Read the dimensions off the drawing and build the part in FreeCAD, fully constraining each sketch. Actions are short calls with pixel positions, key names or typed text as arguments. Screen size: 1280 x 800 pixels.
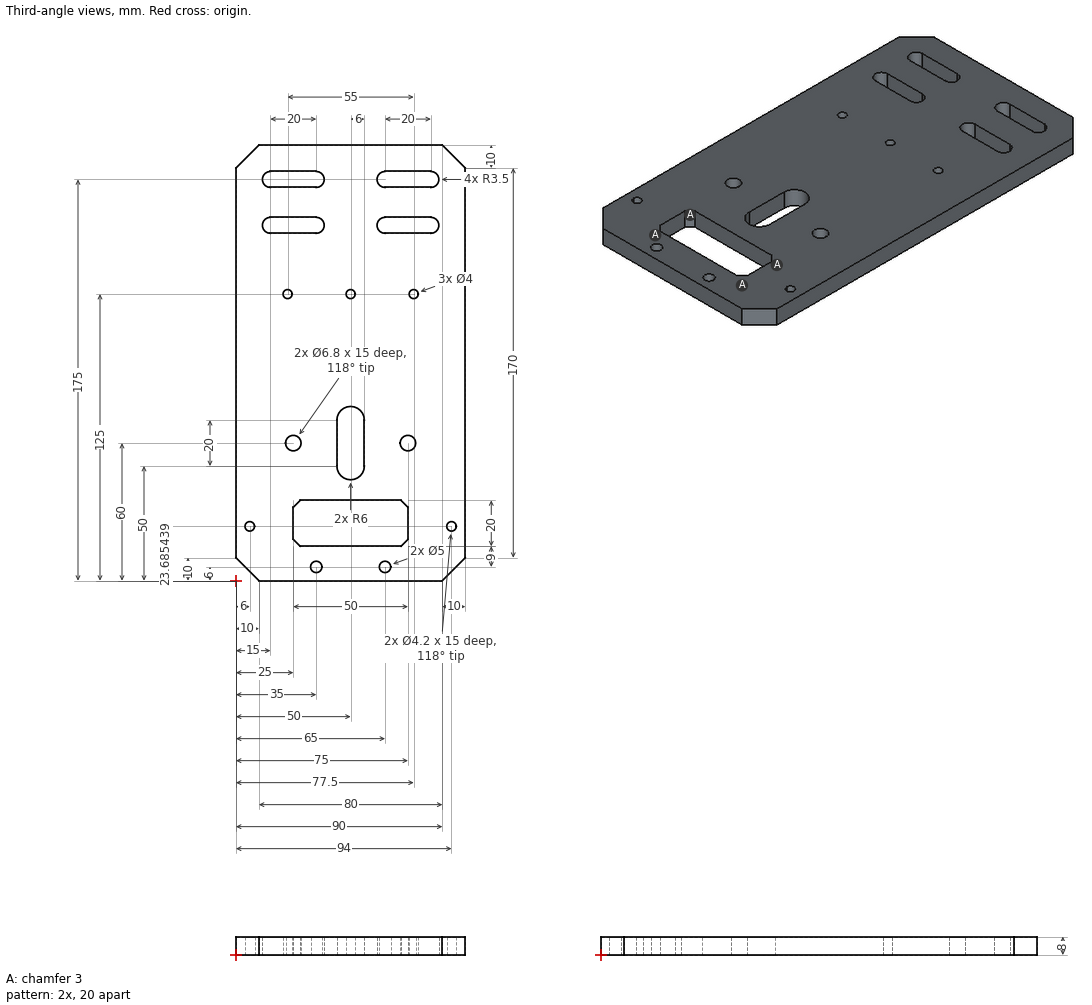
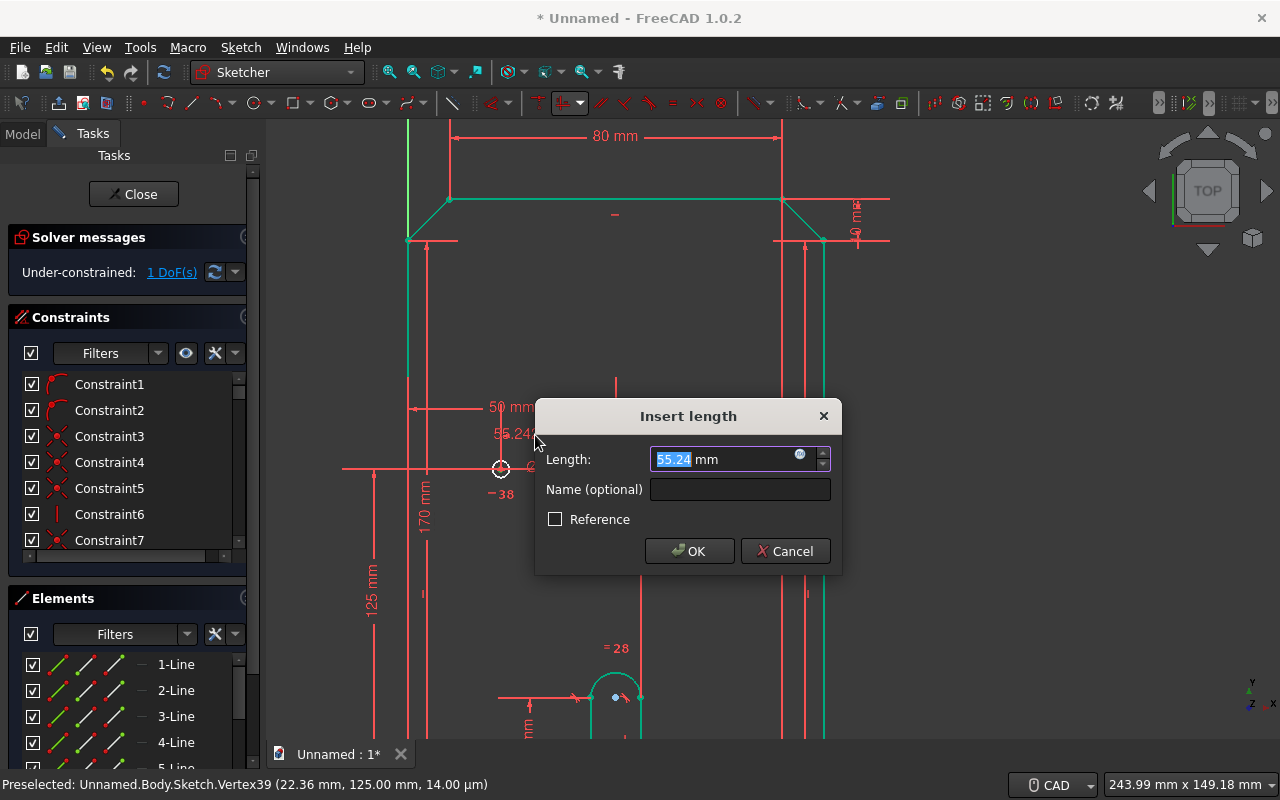
text(55)
key(Return)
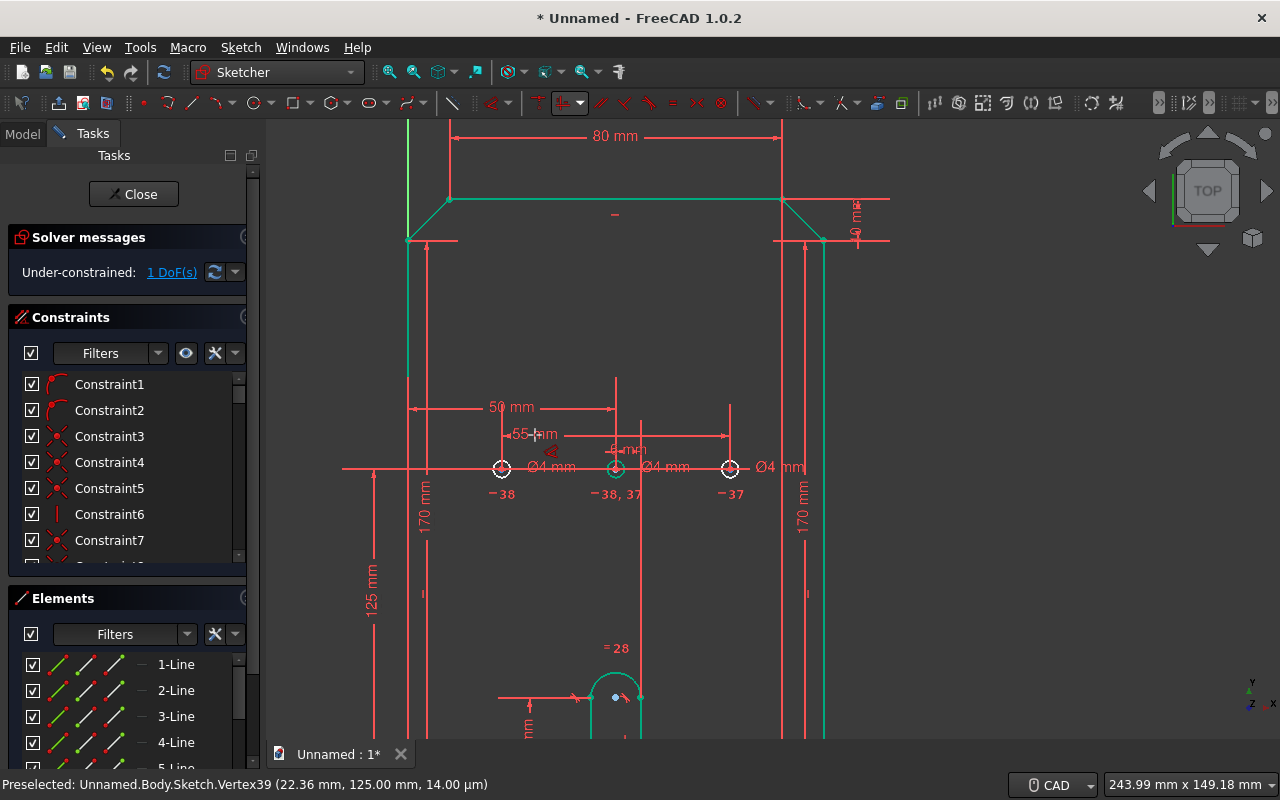
click(730, 469)
click(456, 435)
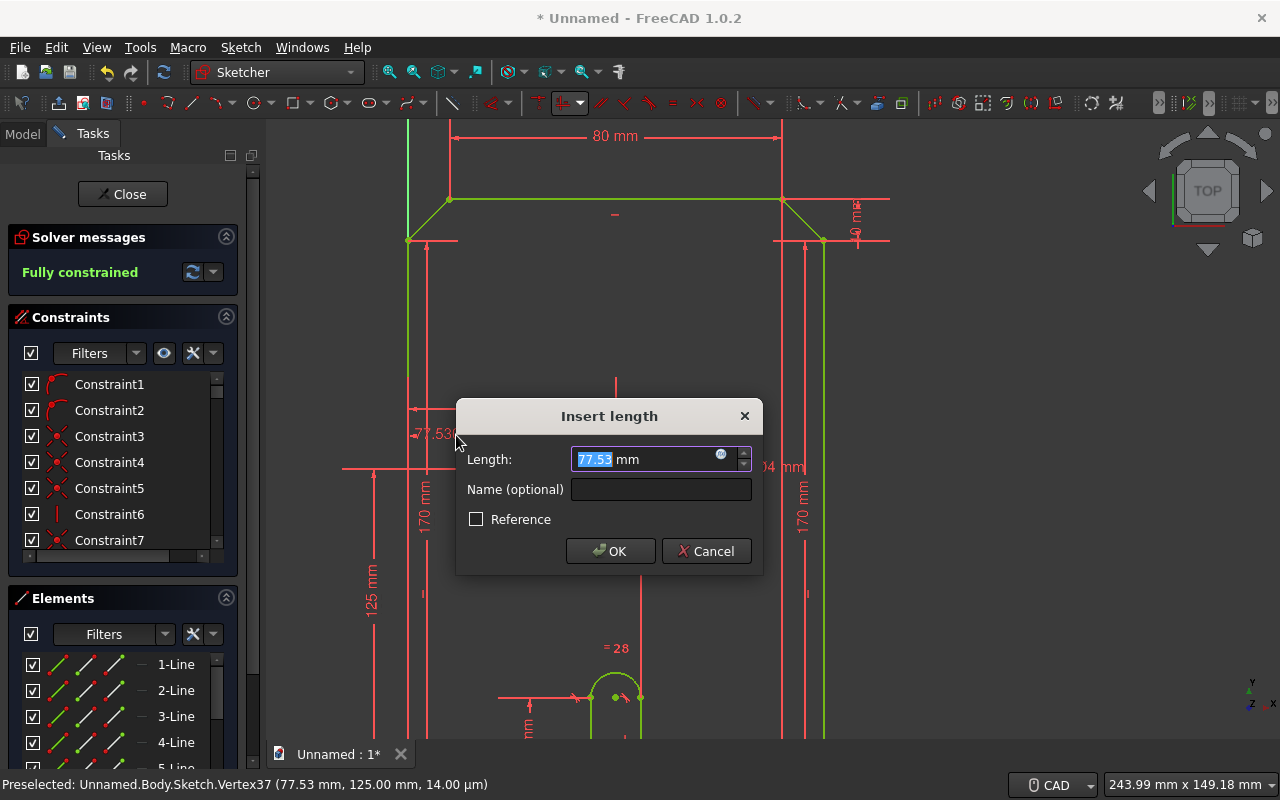
text(77.5)
key(Return)
key(Escape)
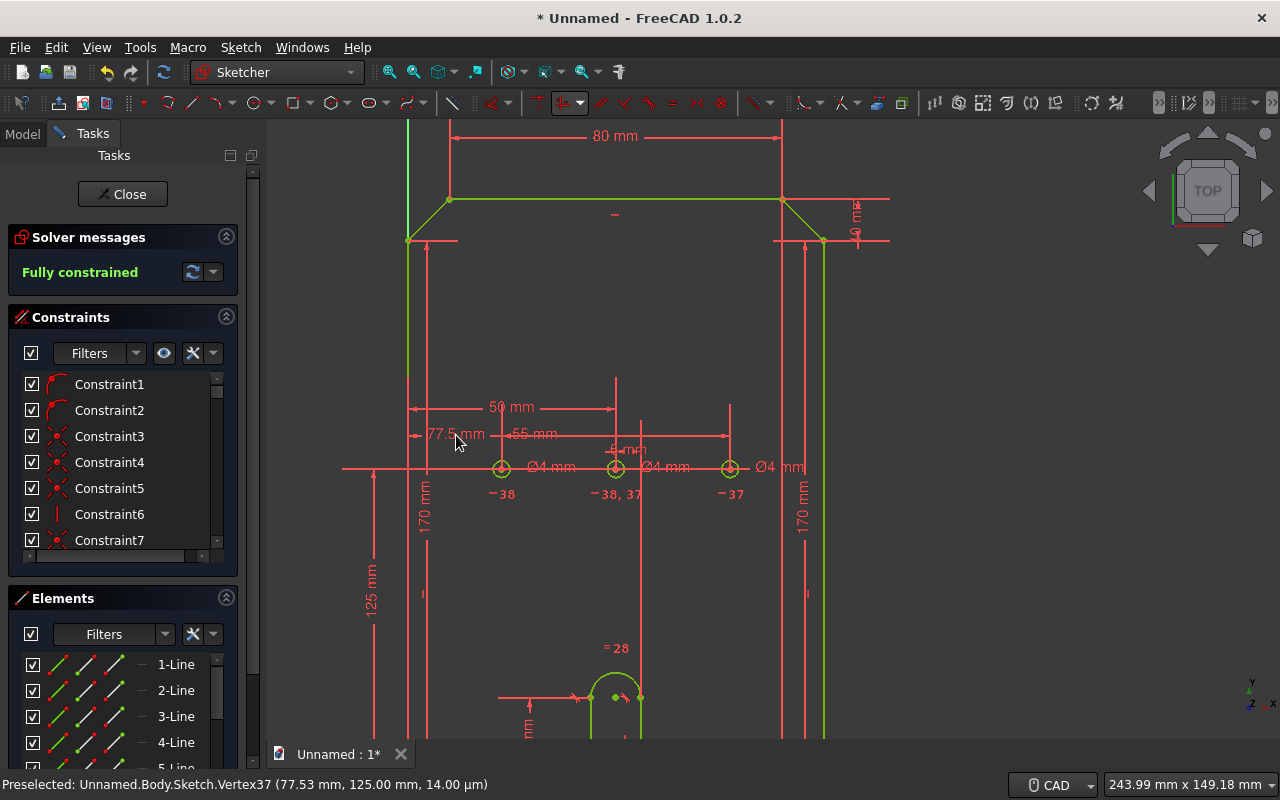
click(123, 194)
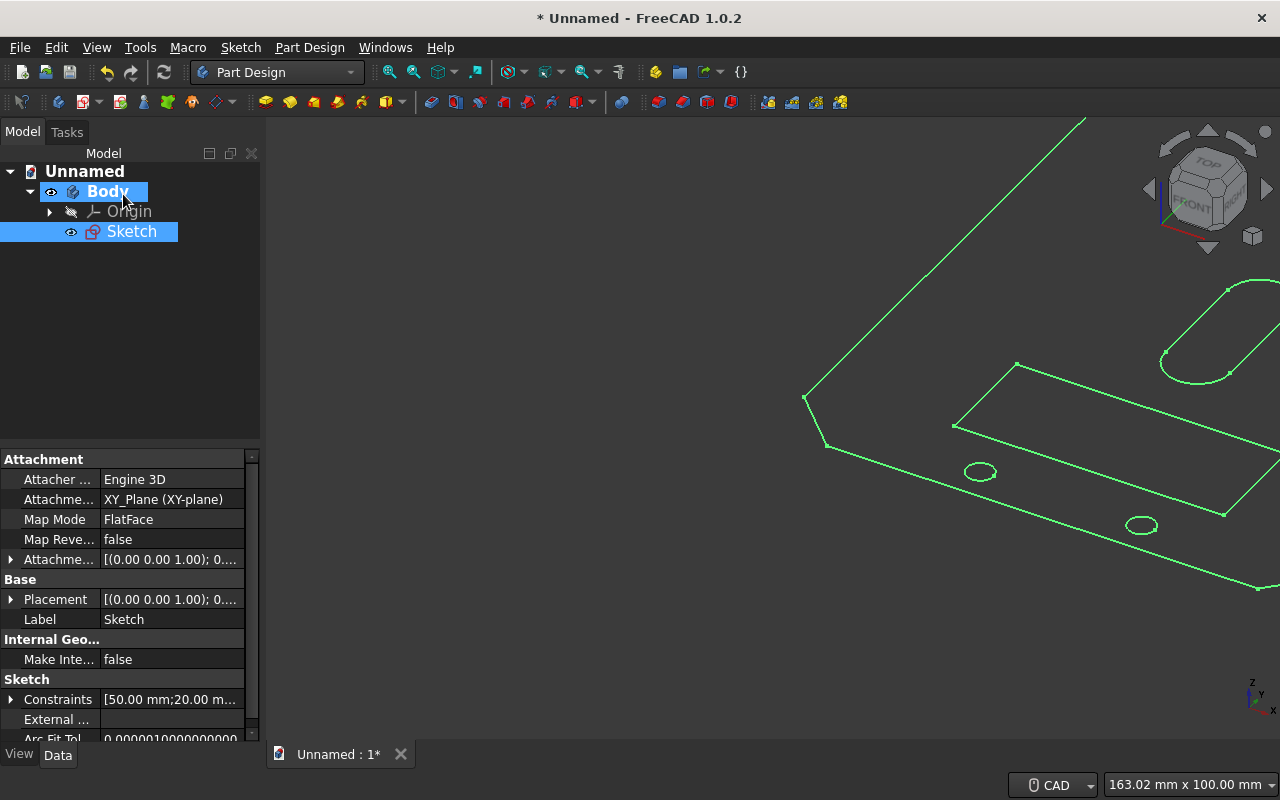
click(266, 102)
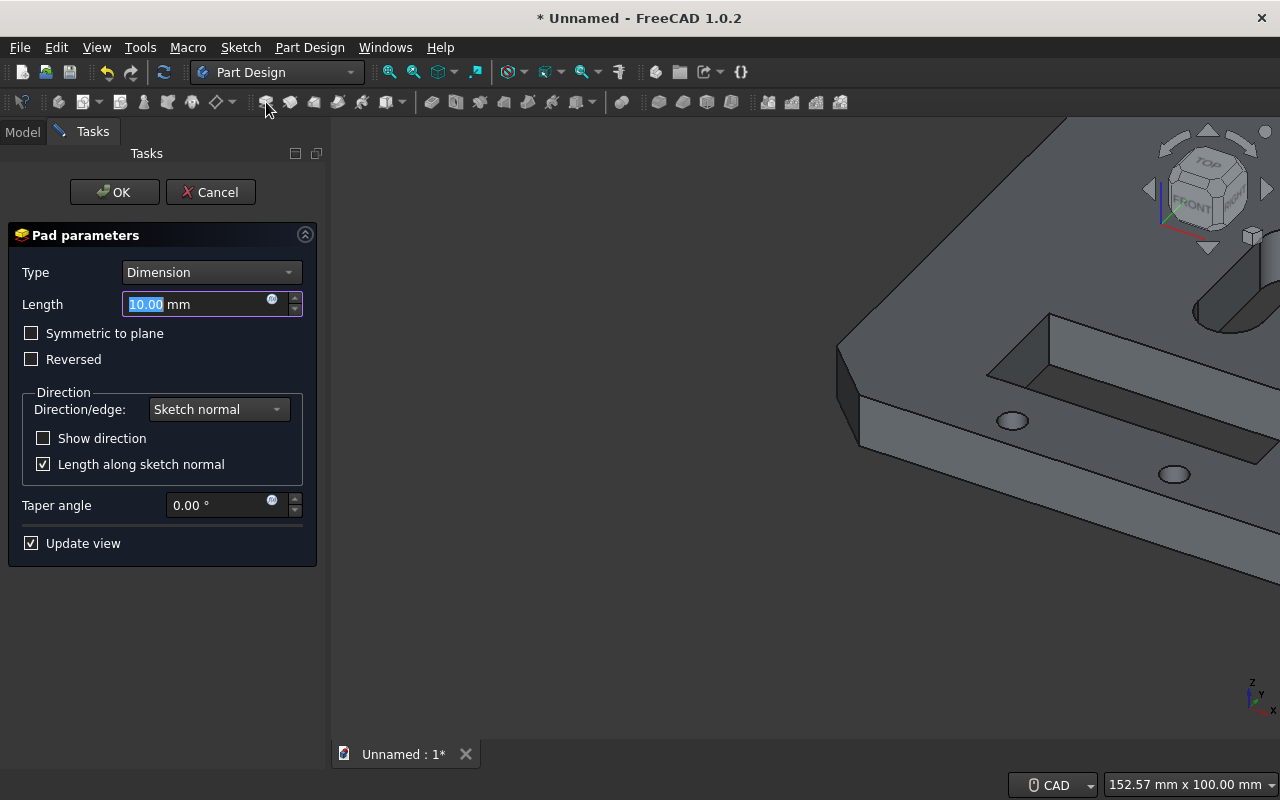
text(8)
key(Tab)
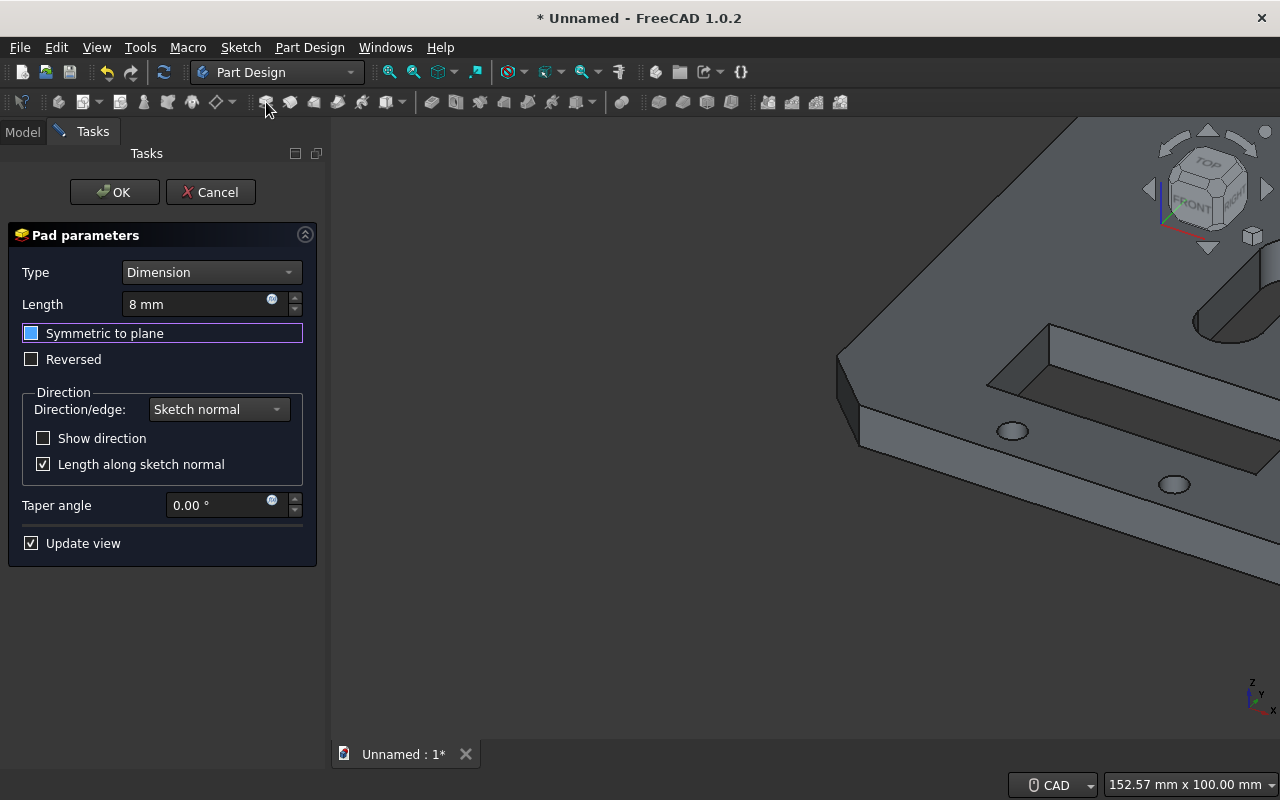
click(115, 192)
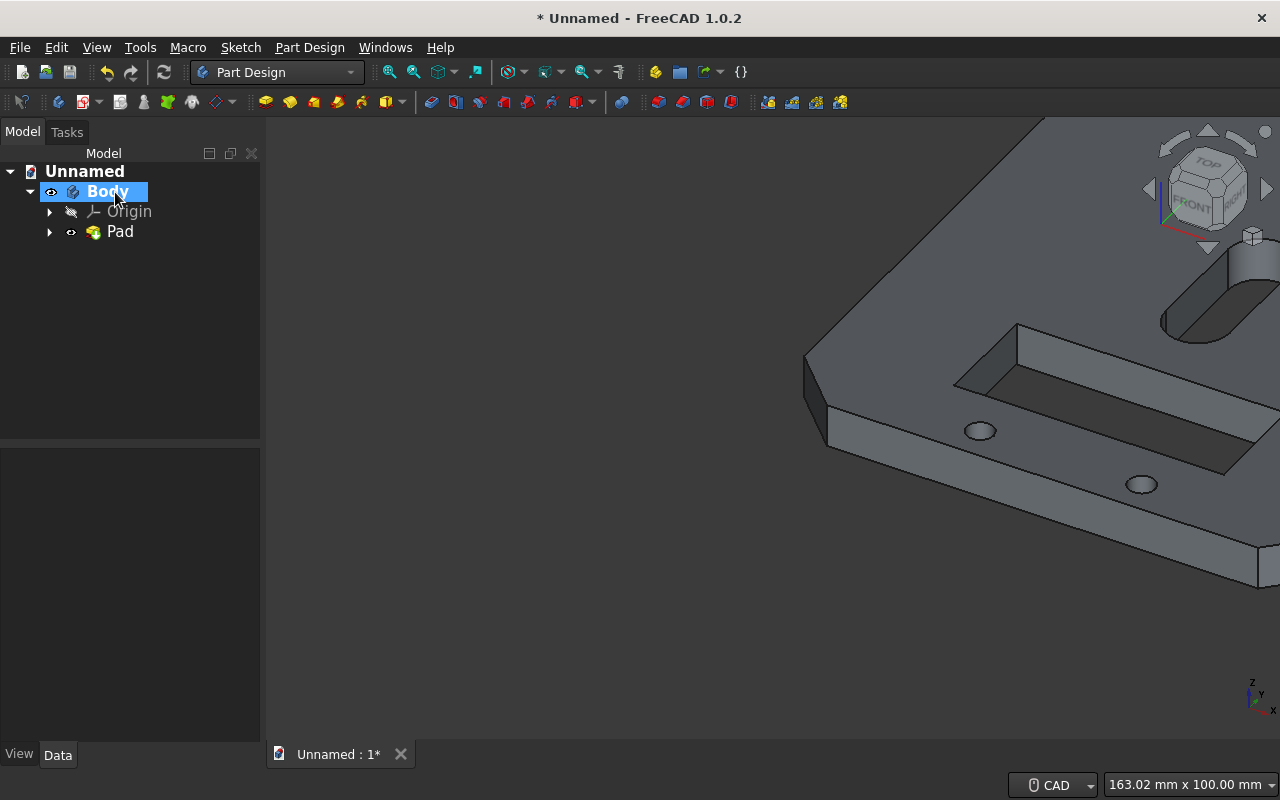
click(390, 72)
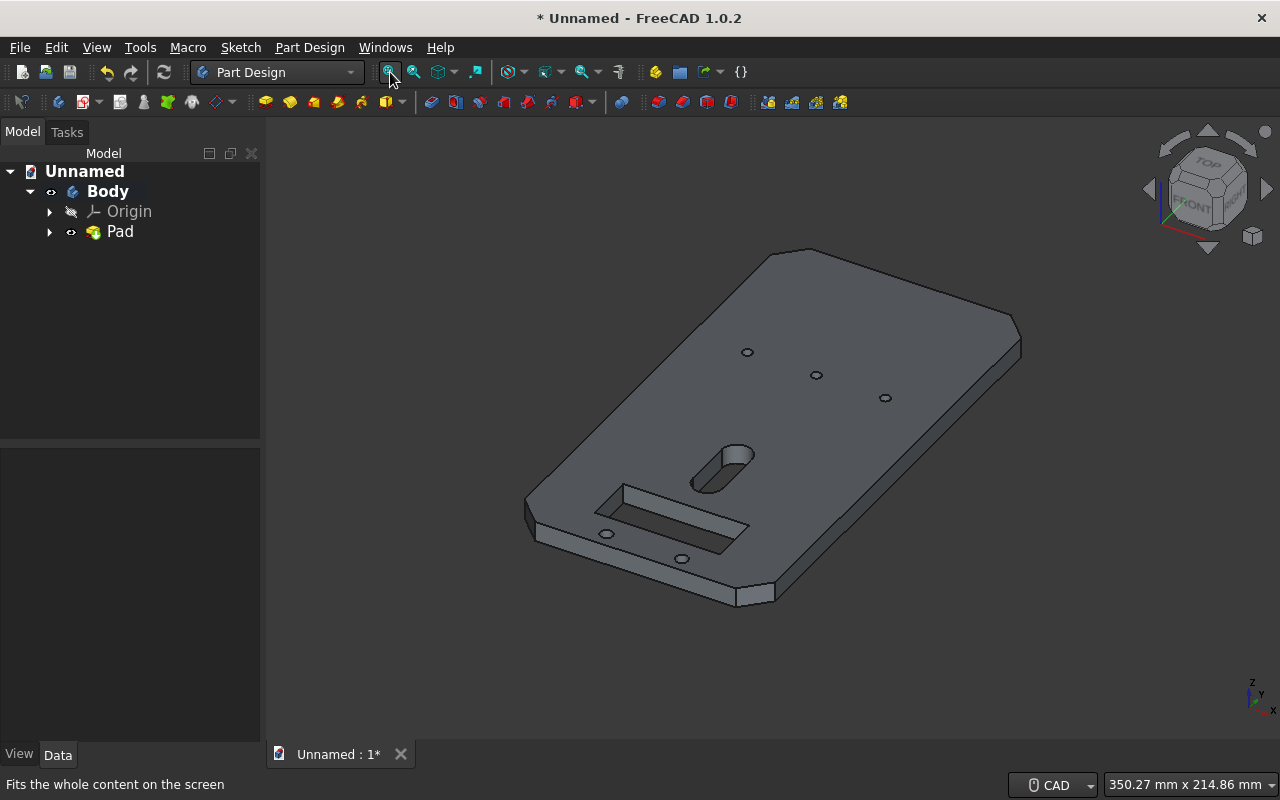
key(0)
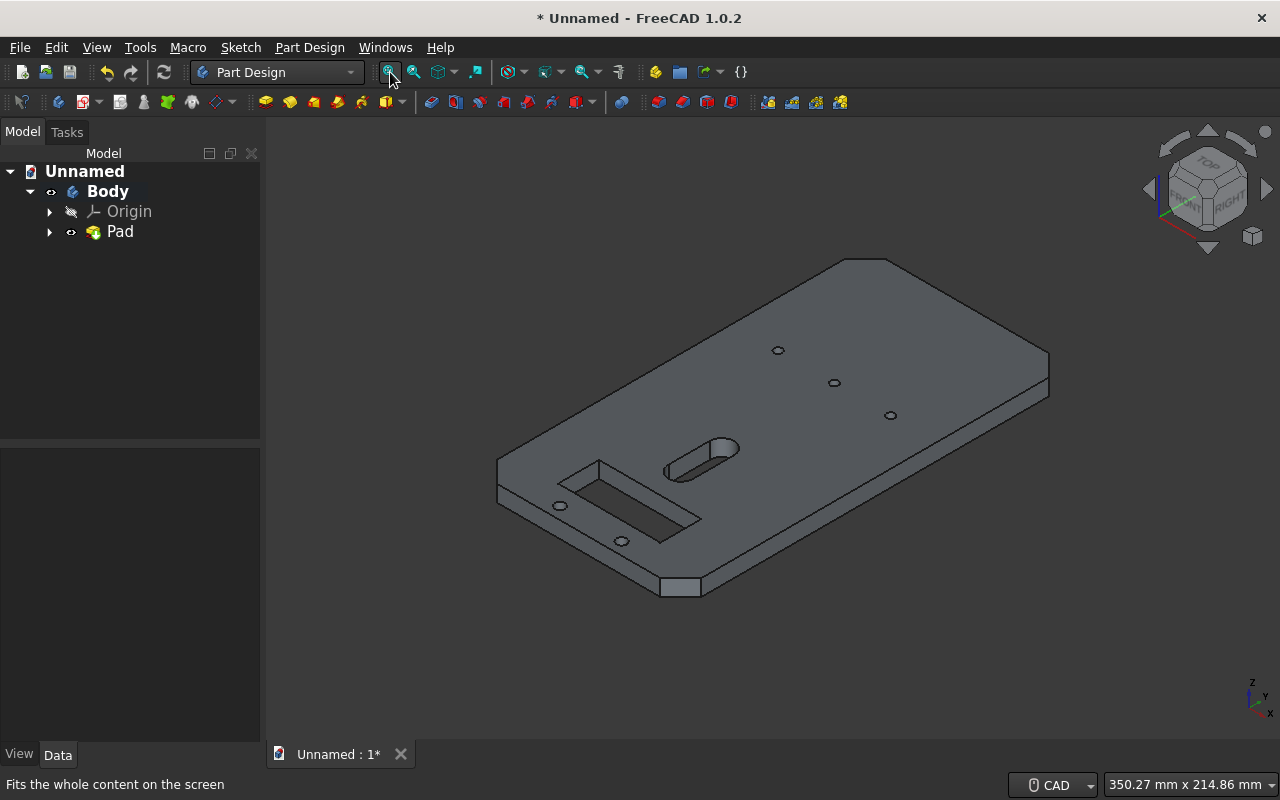
key(2)